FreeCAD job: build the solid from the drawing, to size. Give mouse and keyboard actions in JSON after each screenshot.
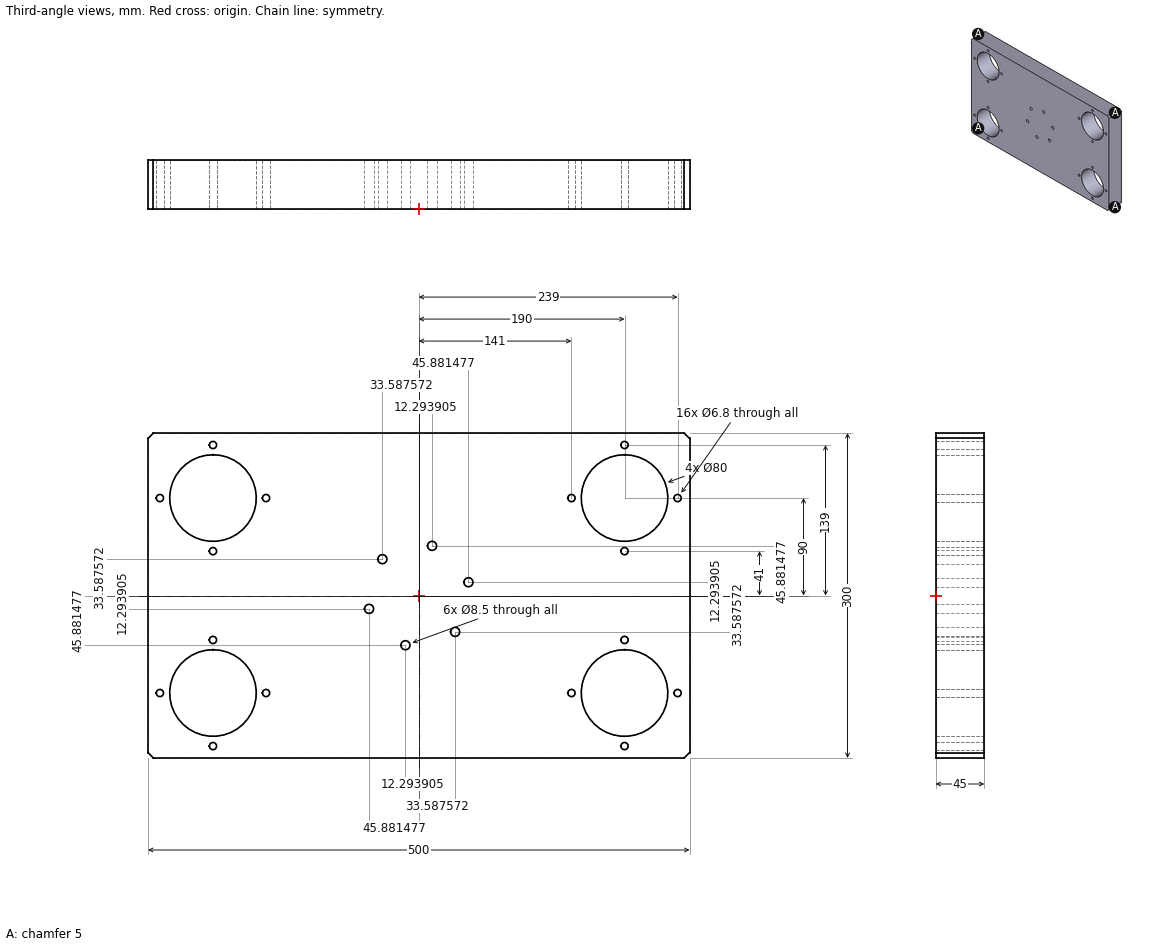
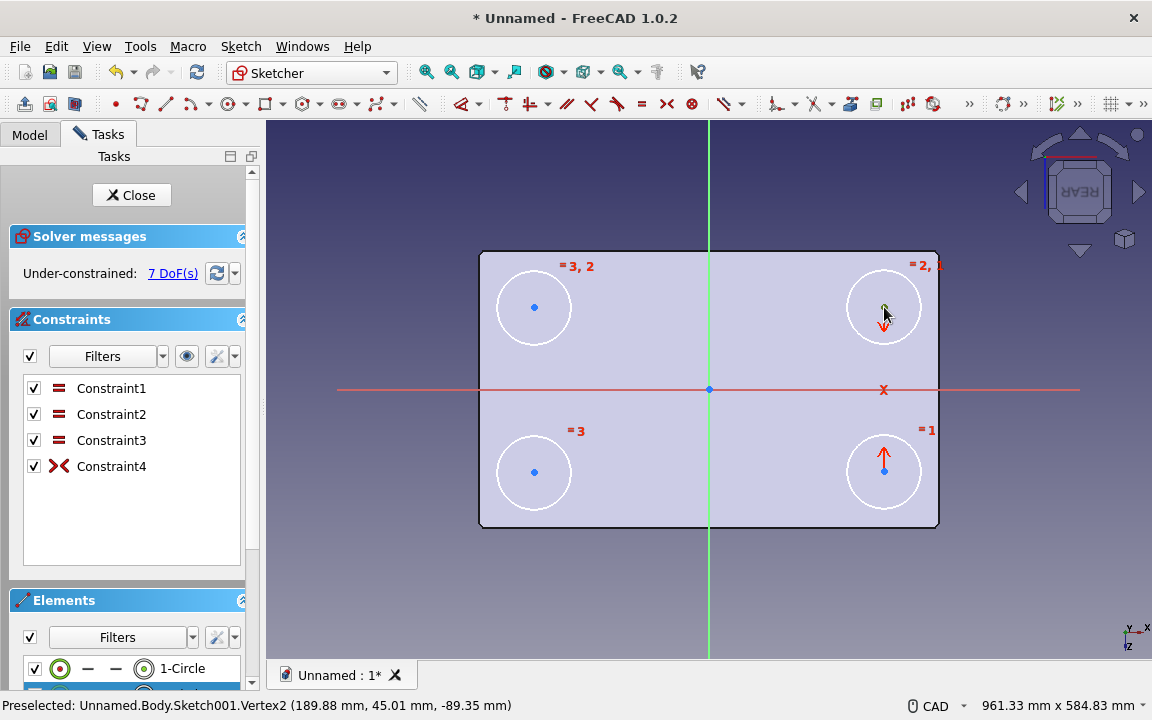
{"action": "left_click", "coordinate": [534, 308]}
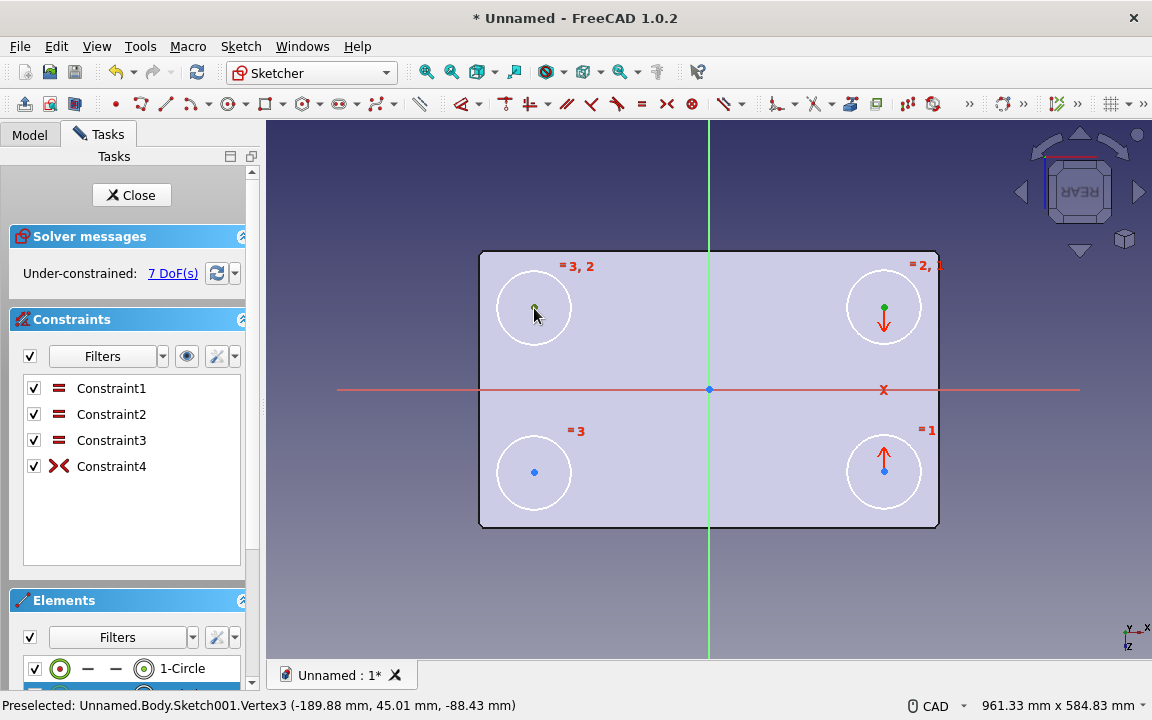
{"action": "left_click", "coordinate": [709, 596]}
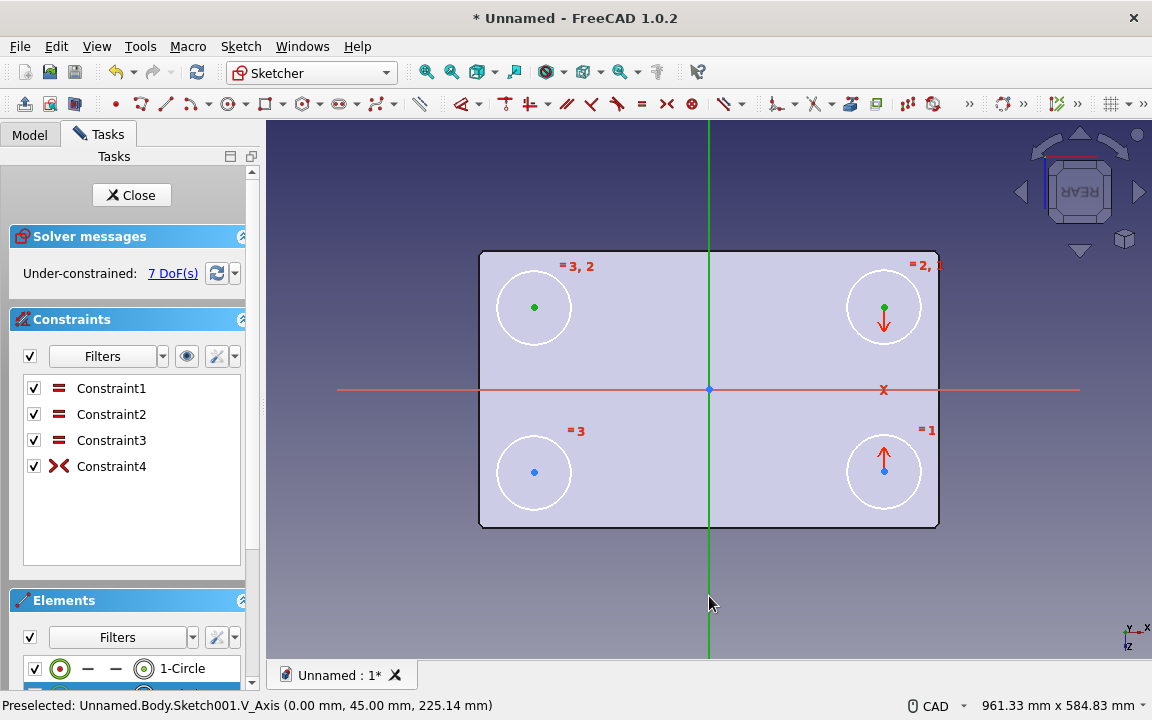
{"action": "left_click", "coordinate": [667, 104]}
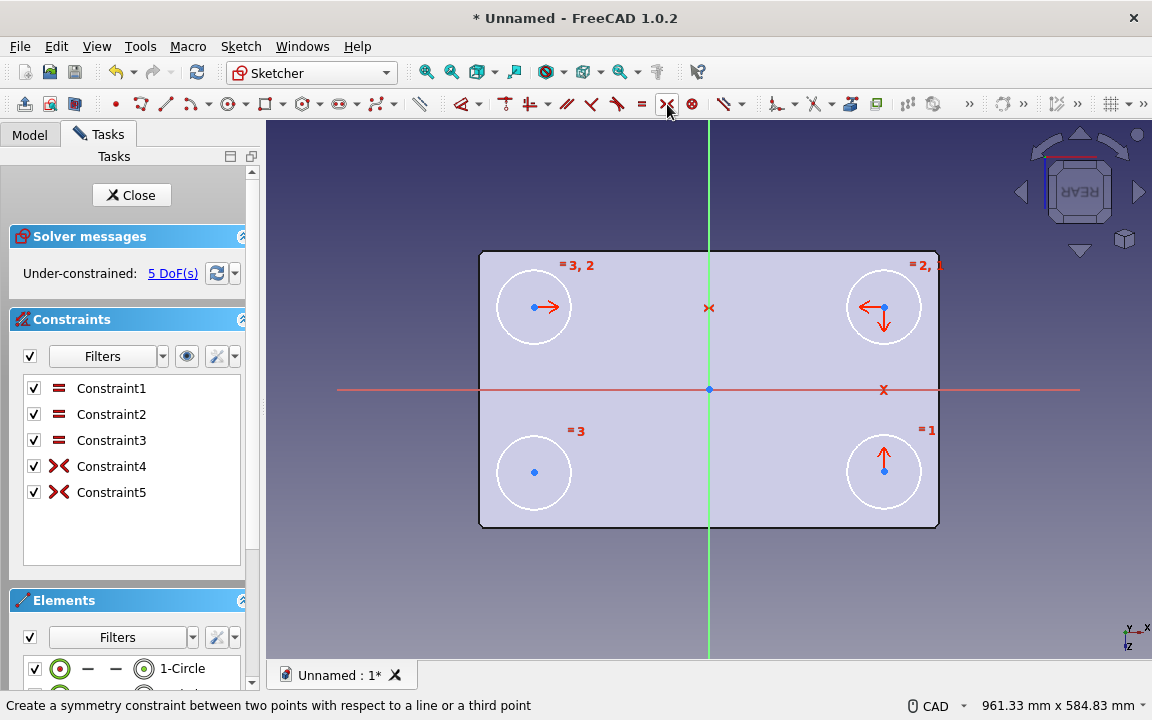
{"action": "left_click", "coordinate": [884, 472]}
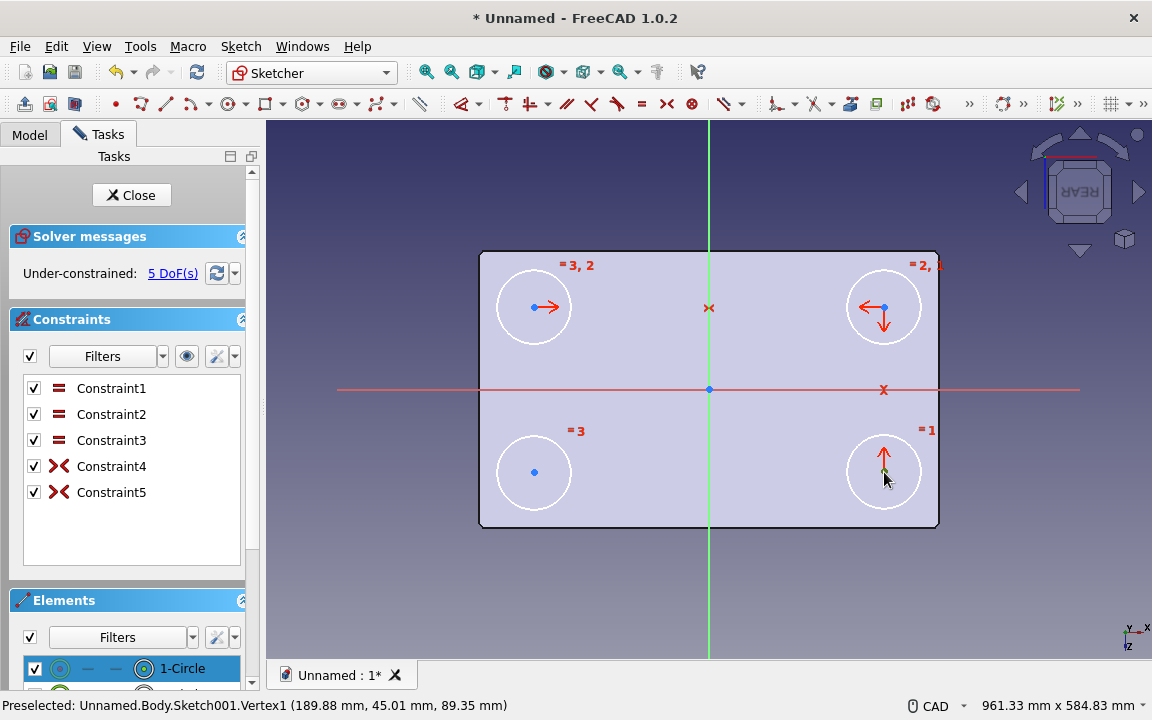
{"action": "left_click", "coordinate": [534, 473]}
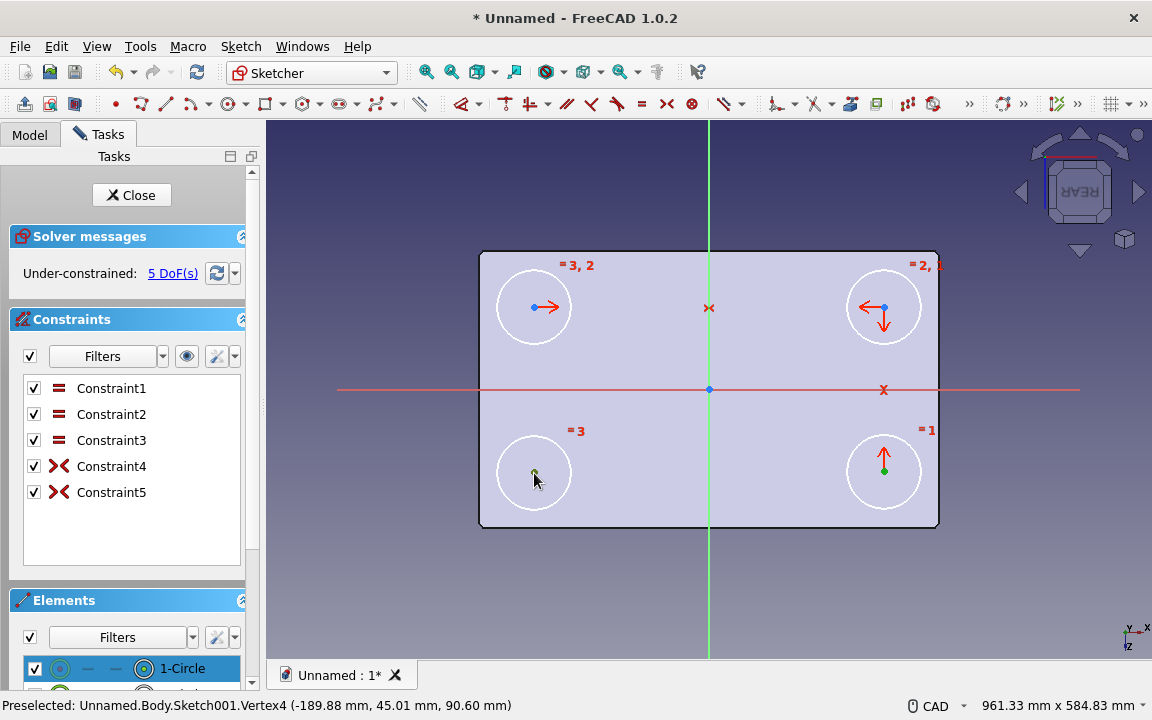
{"action": "left_click", "coordinate": [709, 596]}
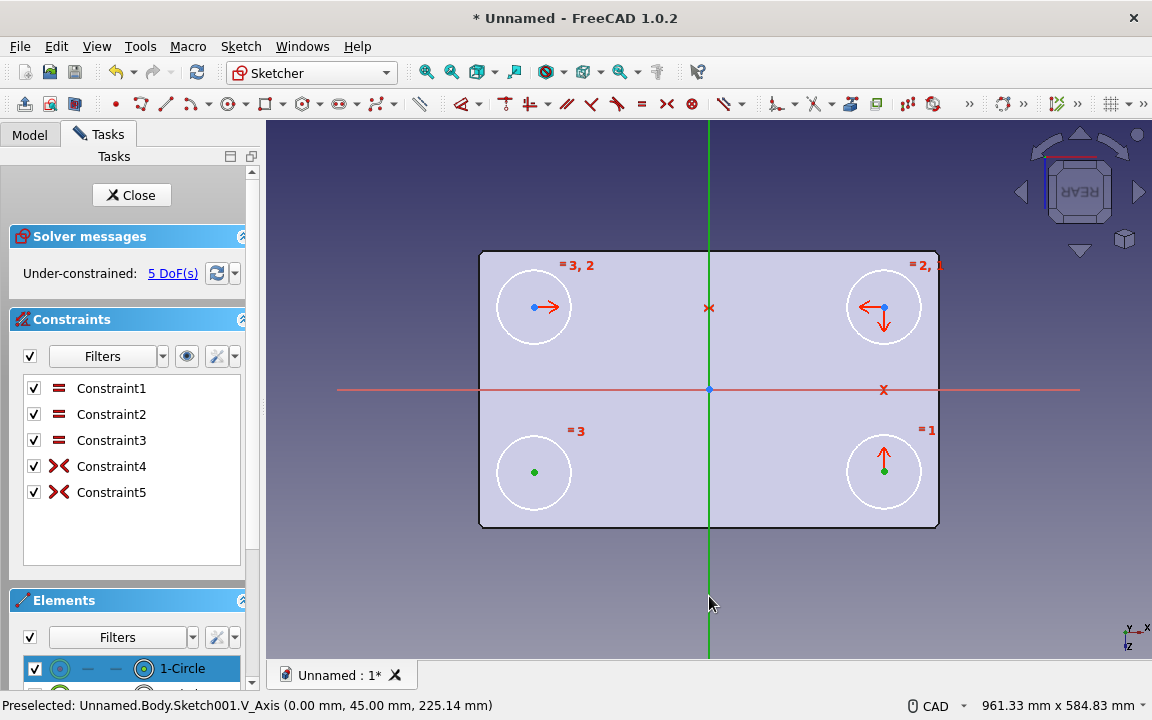
{"action": "left_click", "coordinate": [667, 104]}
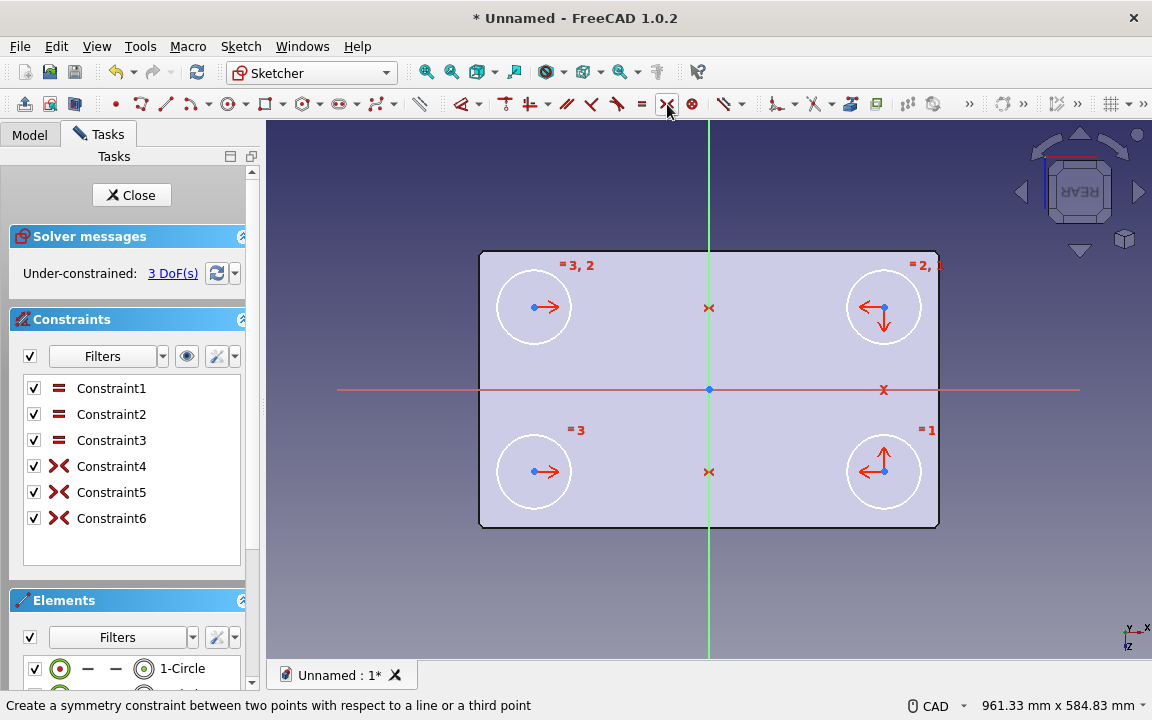
{"action": "left_click", "coordinate": [460, 104]}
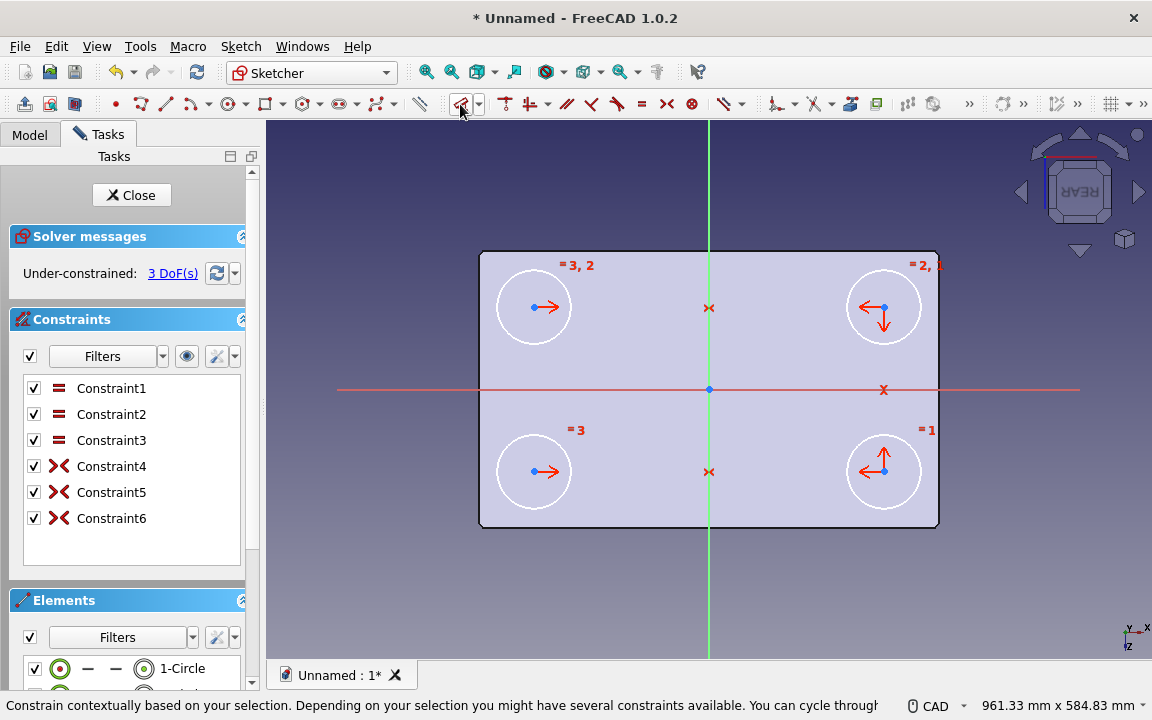
{"action": "left_click", "coordinate": [910, 446]}
{"action": "left_click", "coordinate": [933, 423]}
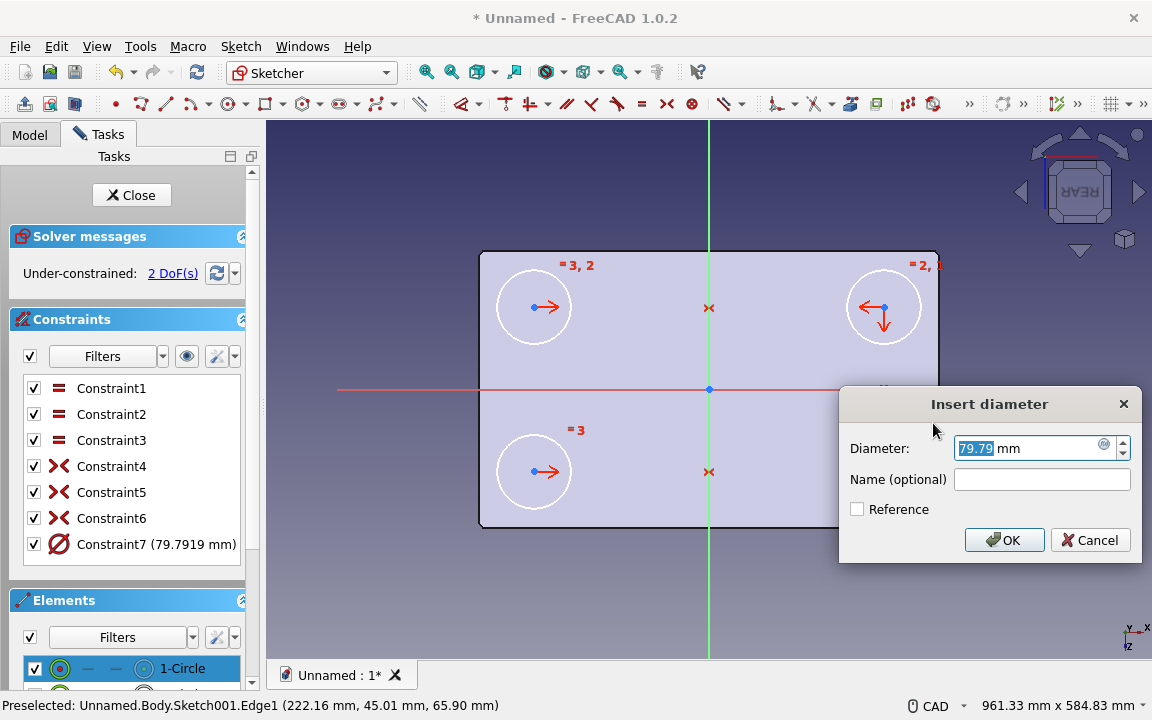
{"action": "type", "text": "80"}
{"action": "key", "text": "Return"}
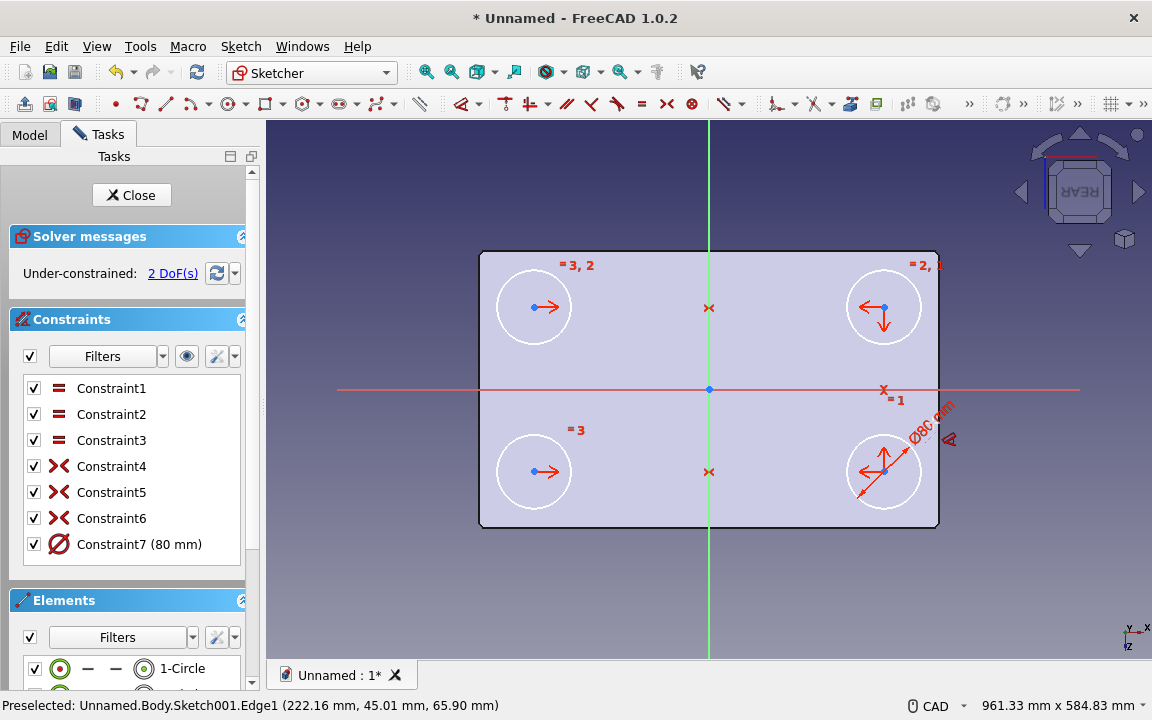
{"action": "left_click", "coordinate": [884, 472]}
{"action": "left_click", "coordinate": [675, 431]}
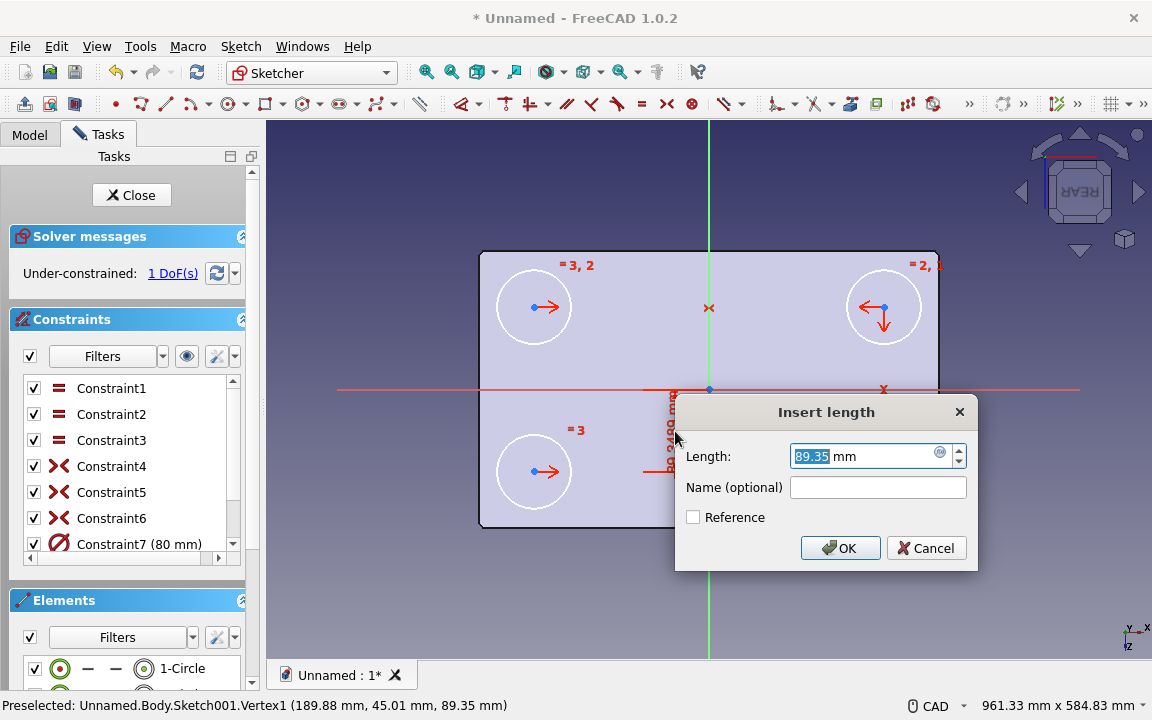
{"action": "type", "text": "90"}
{"action": "key", "text": "Return"}